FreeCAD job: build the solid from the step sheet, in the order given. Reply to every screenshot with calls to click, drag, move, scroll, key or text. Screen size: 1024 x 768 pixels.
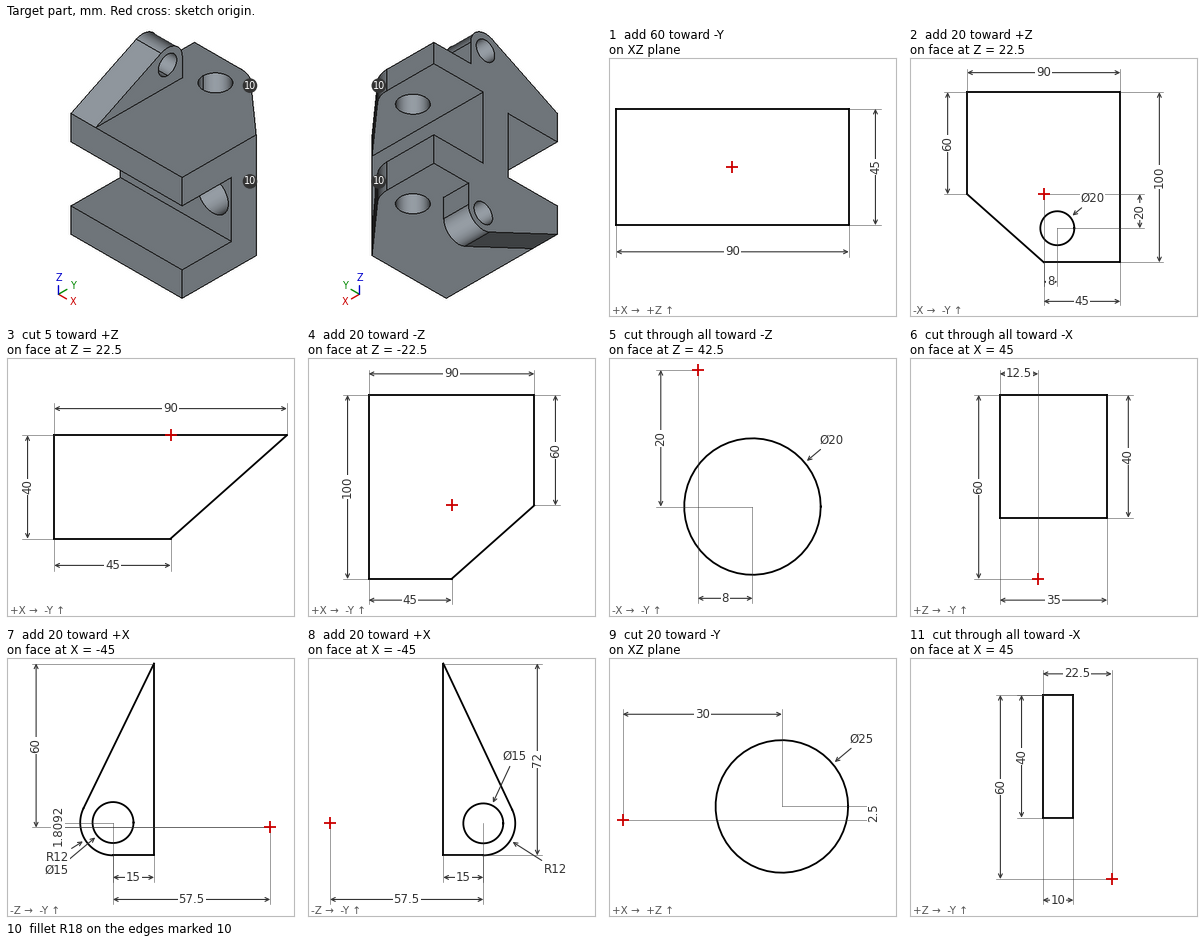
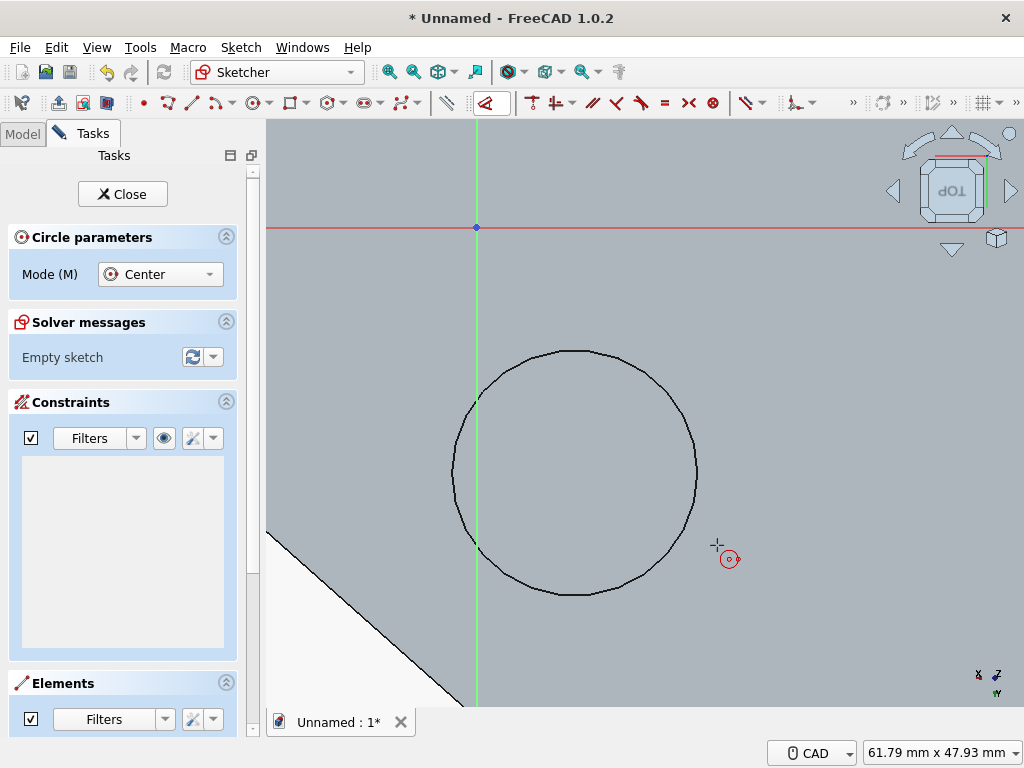
click(575, 473)
move(661, 386)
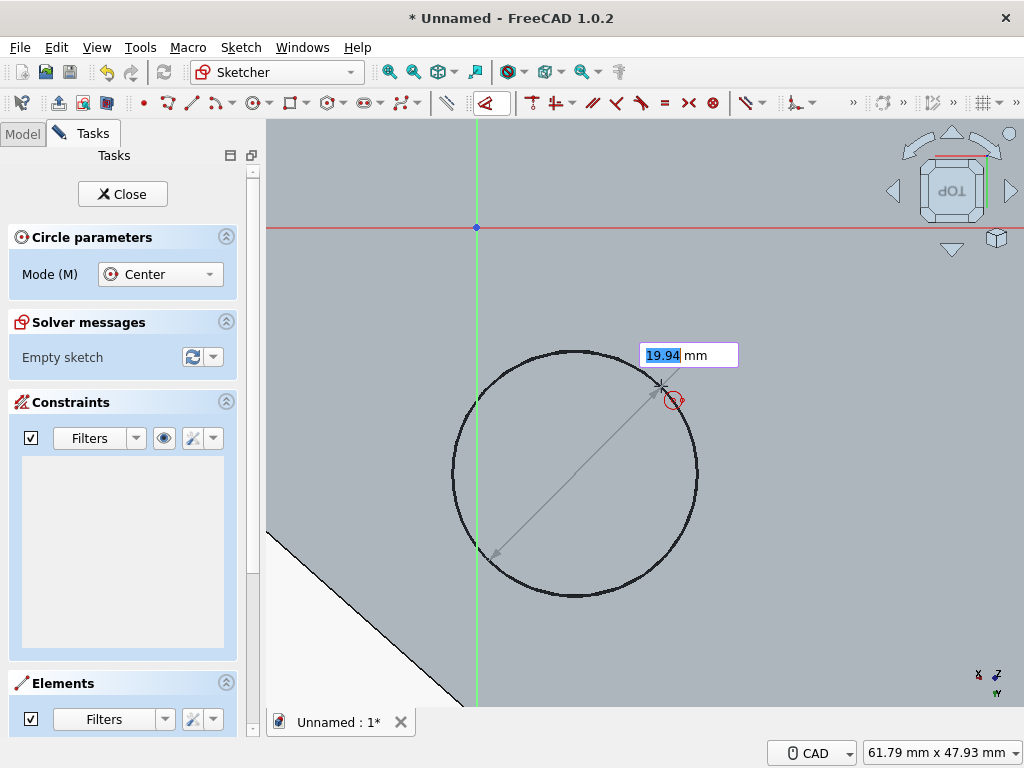
text(20)
key(Return)
key(Escape)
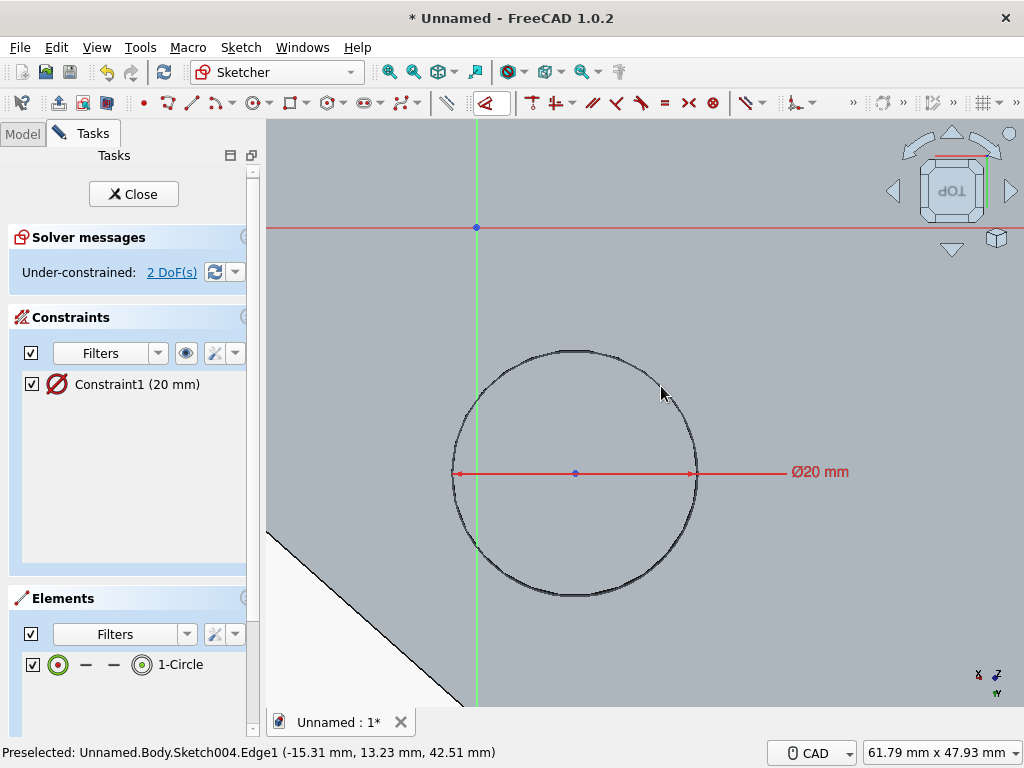
click(575, 474)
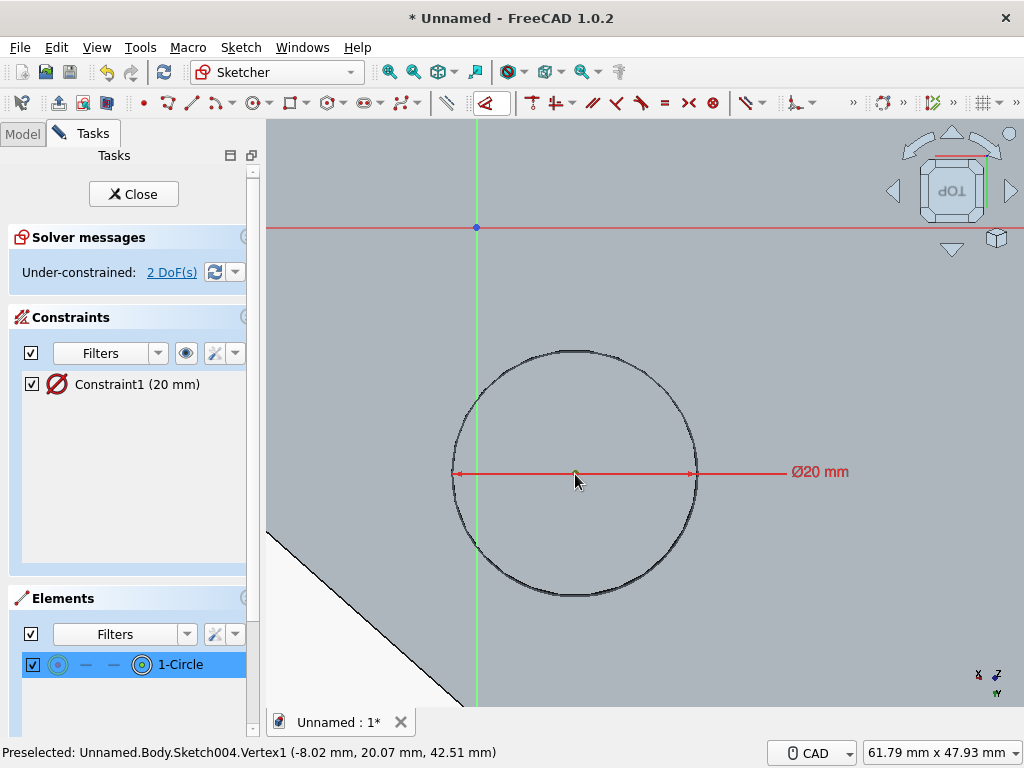
click(504, 104)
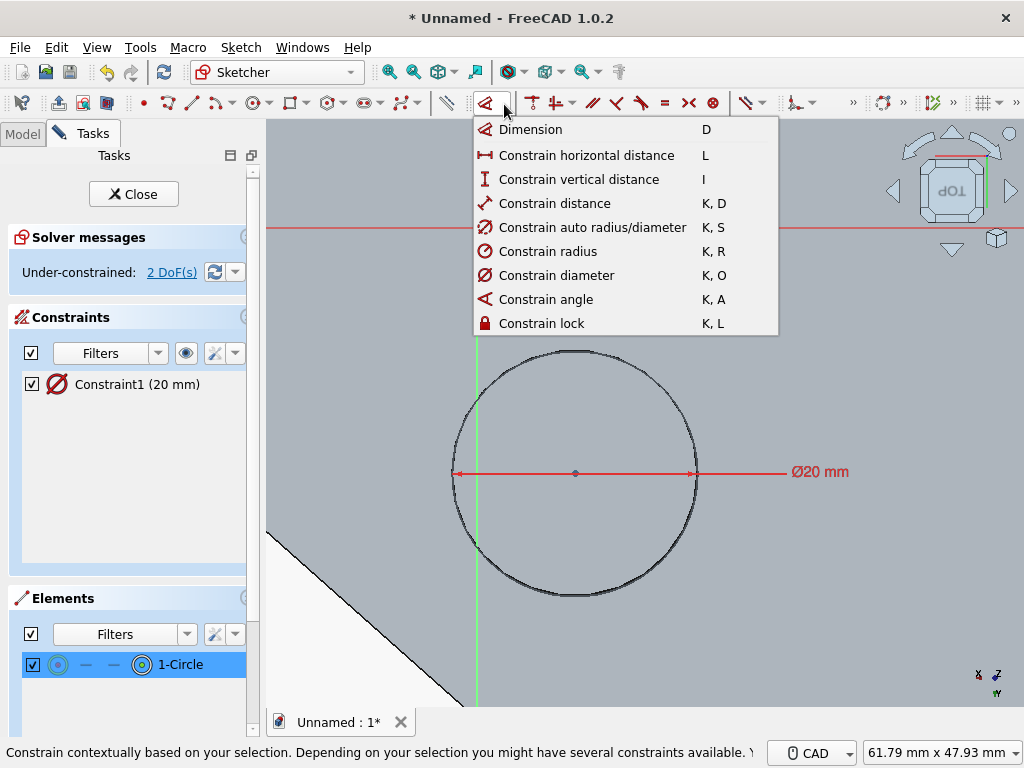
click(626, 155)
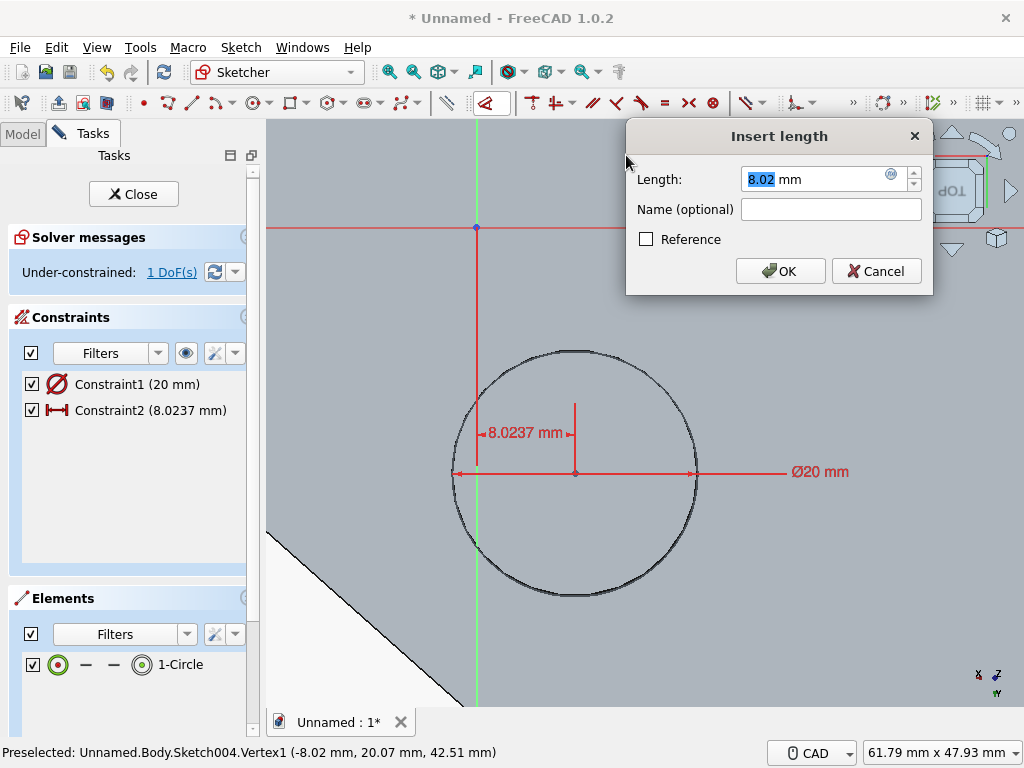
text(8)
key(Return)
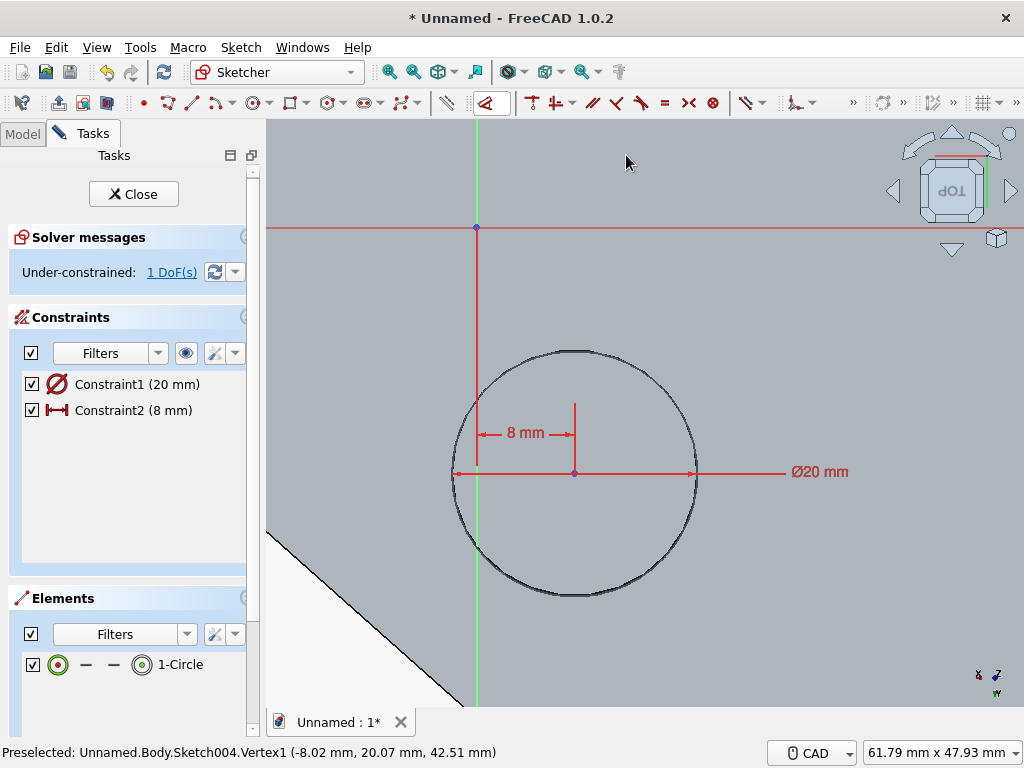
click(575, 474)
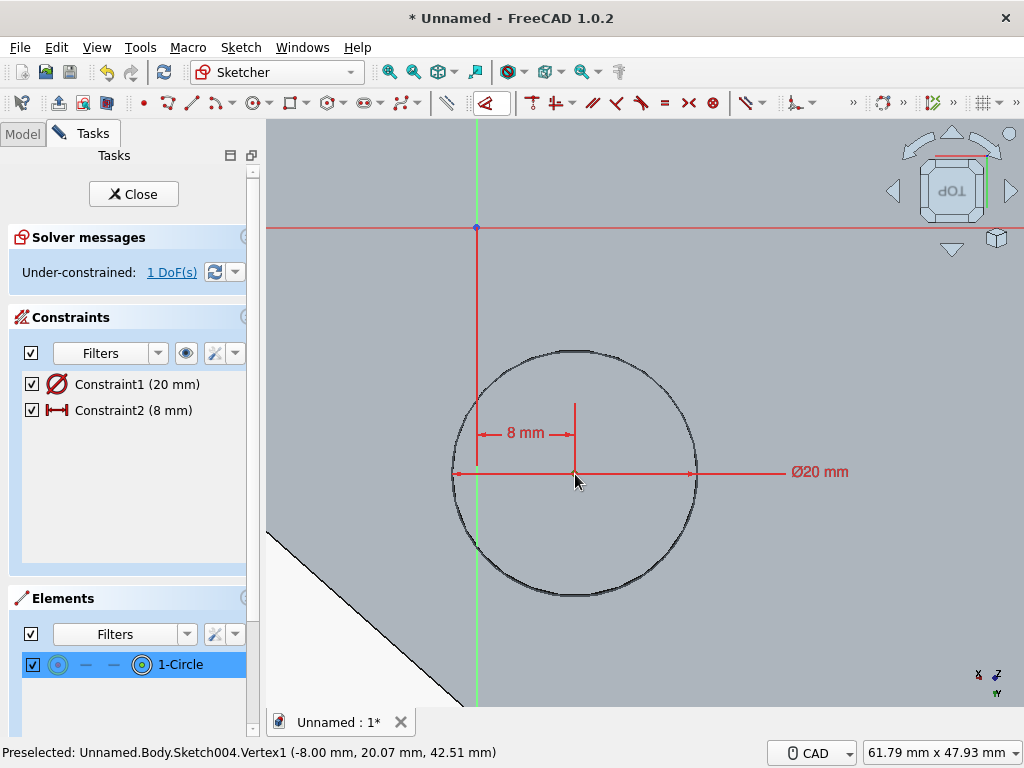
key(i)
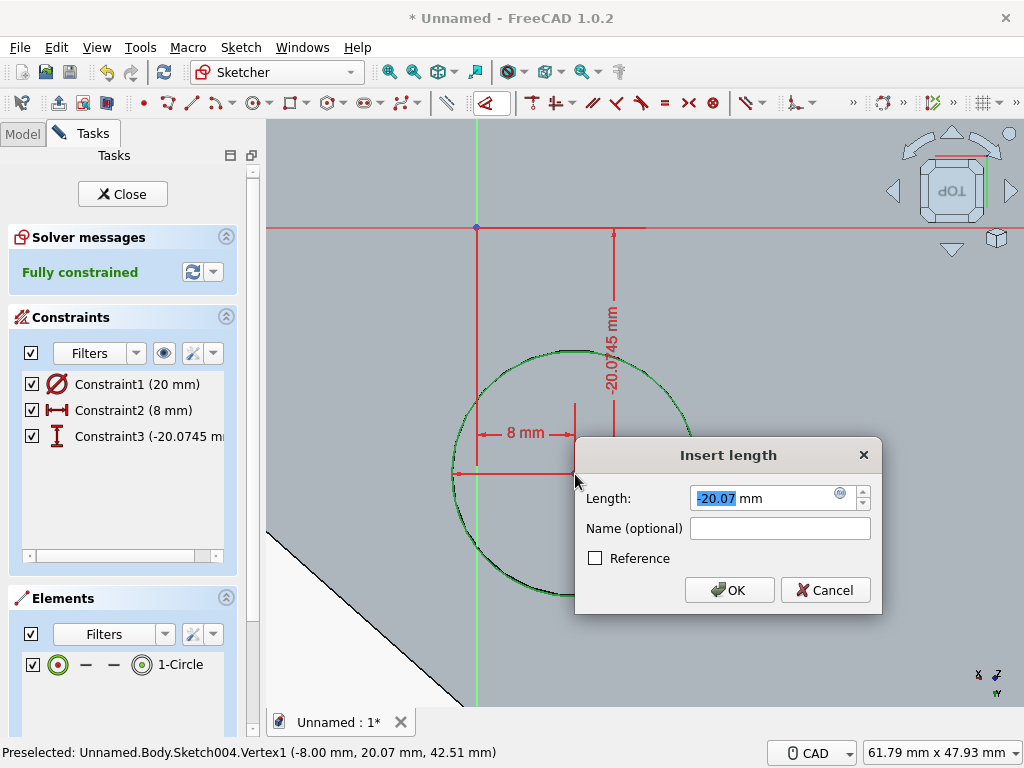
text(-20)
key(Return)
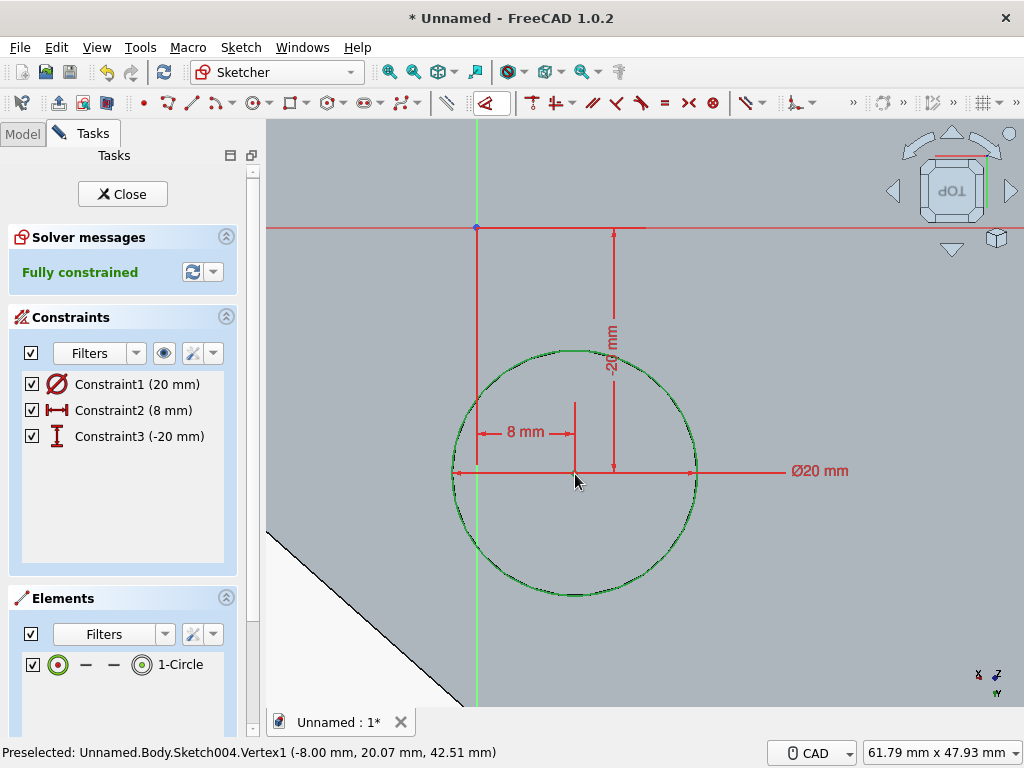
click(123, 194)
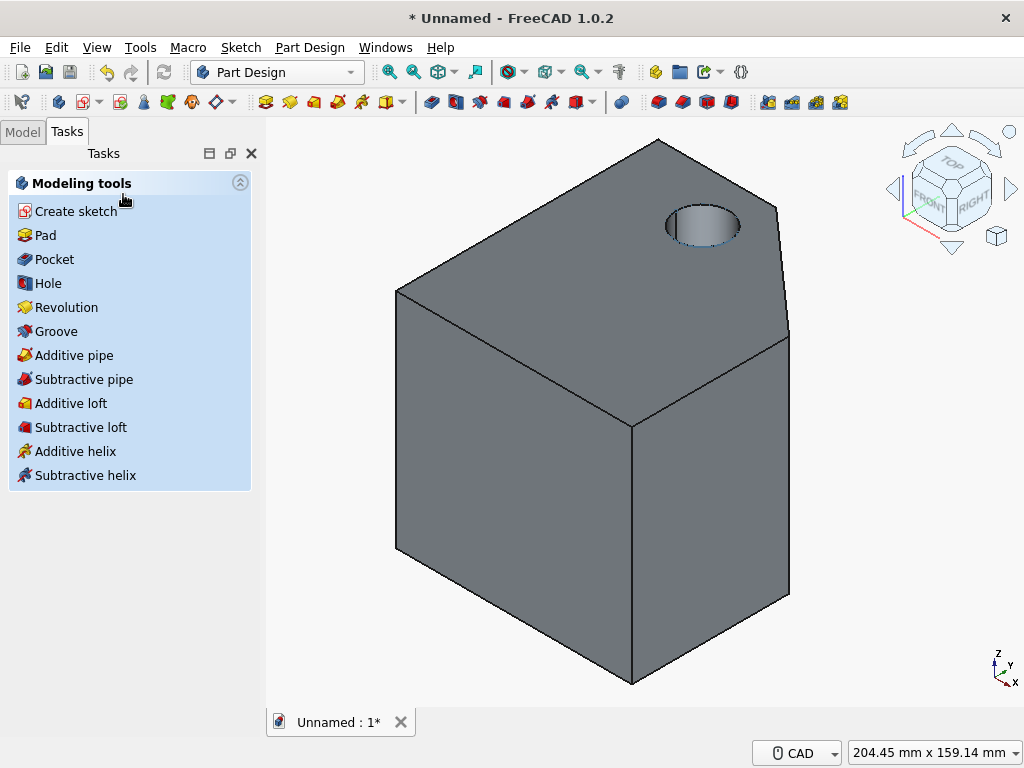
click(432, 102)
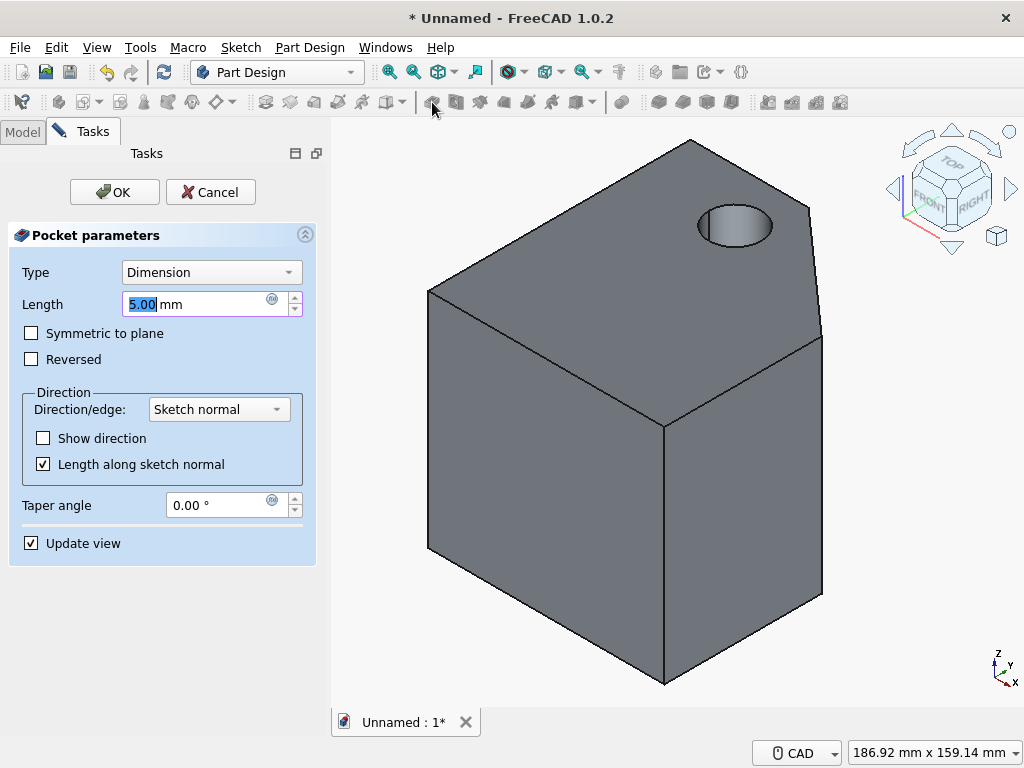
click(212, 272)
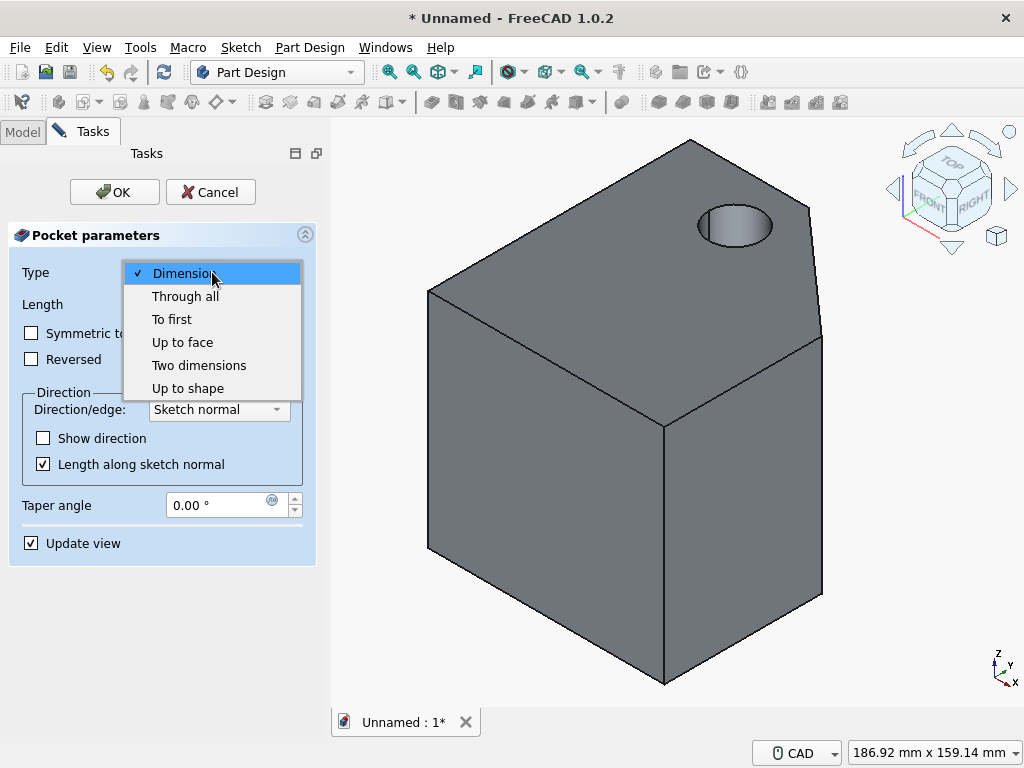
click(212, 296)